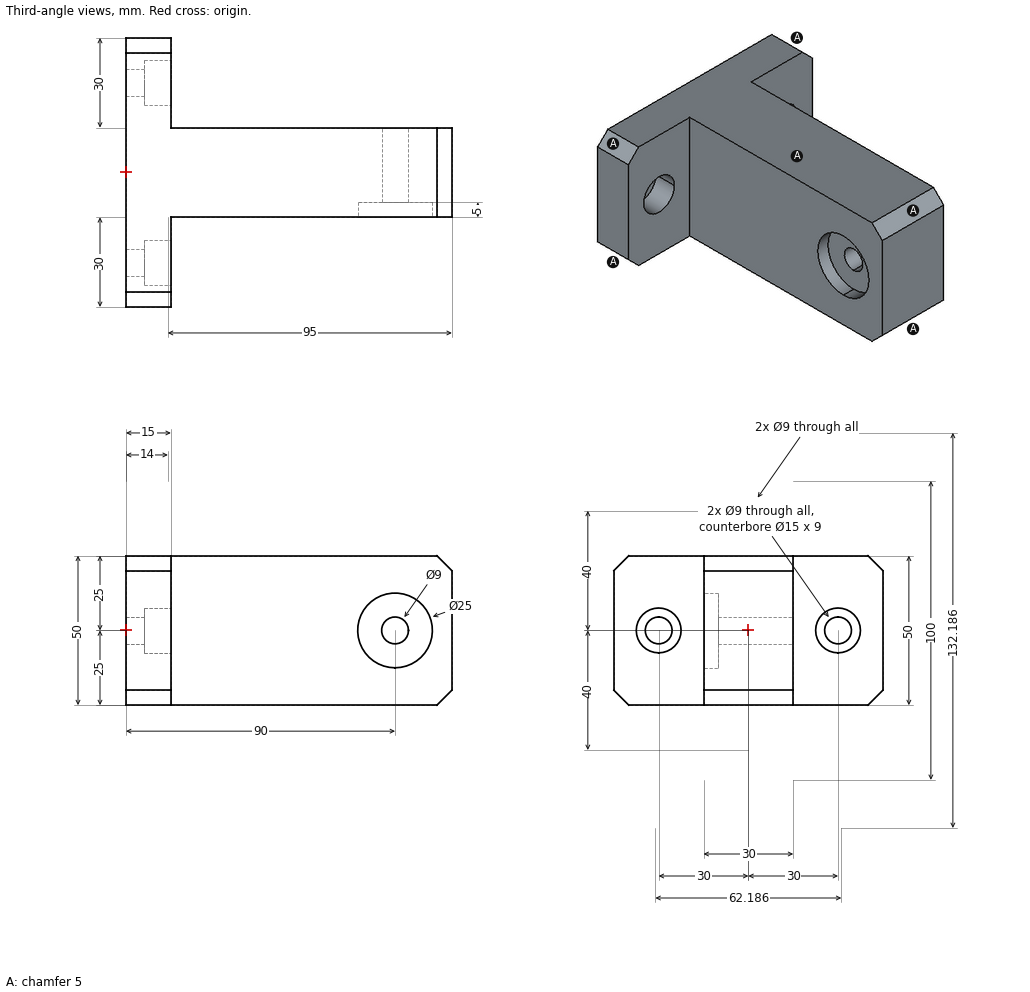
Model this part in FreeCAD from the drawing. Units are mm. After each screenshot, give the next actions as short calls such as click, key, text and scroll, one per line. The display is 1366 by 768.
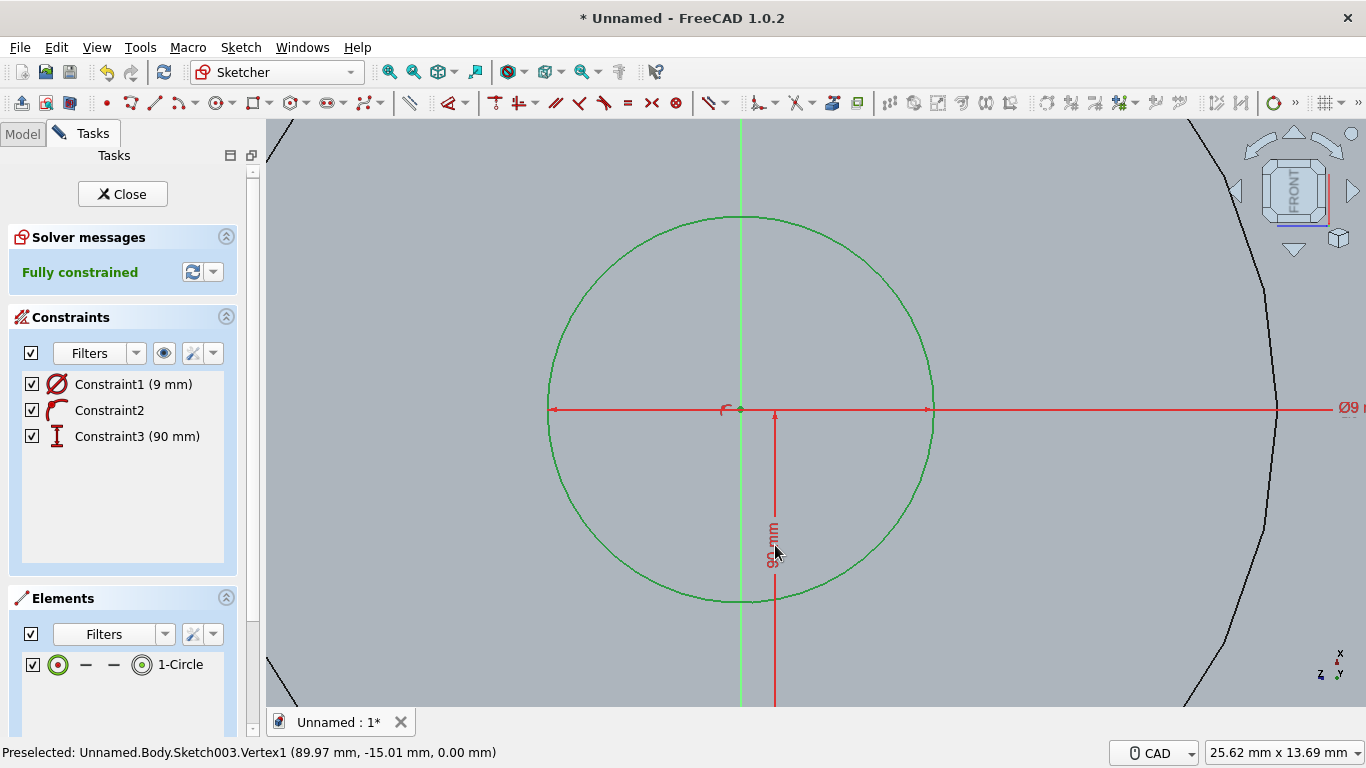
click(123, 194)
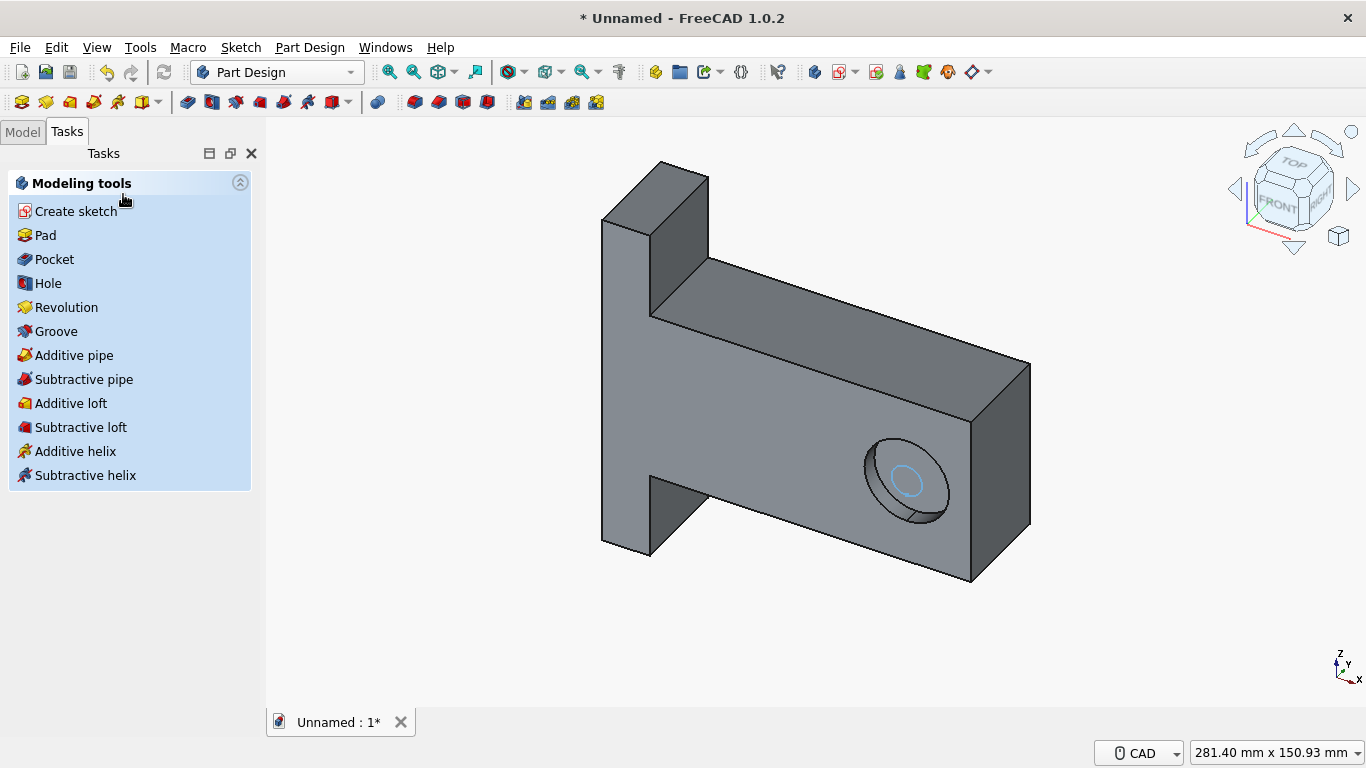
click(188, 102)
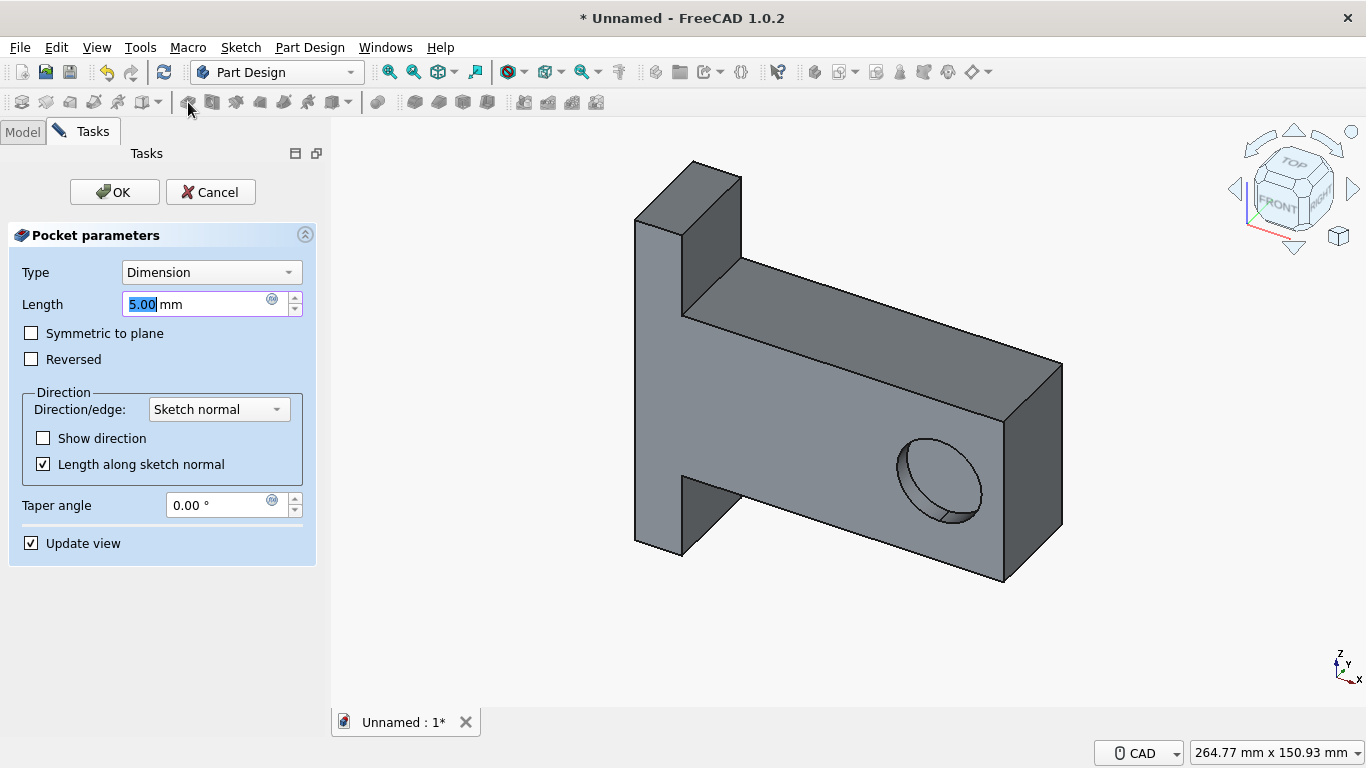
click(212, 272)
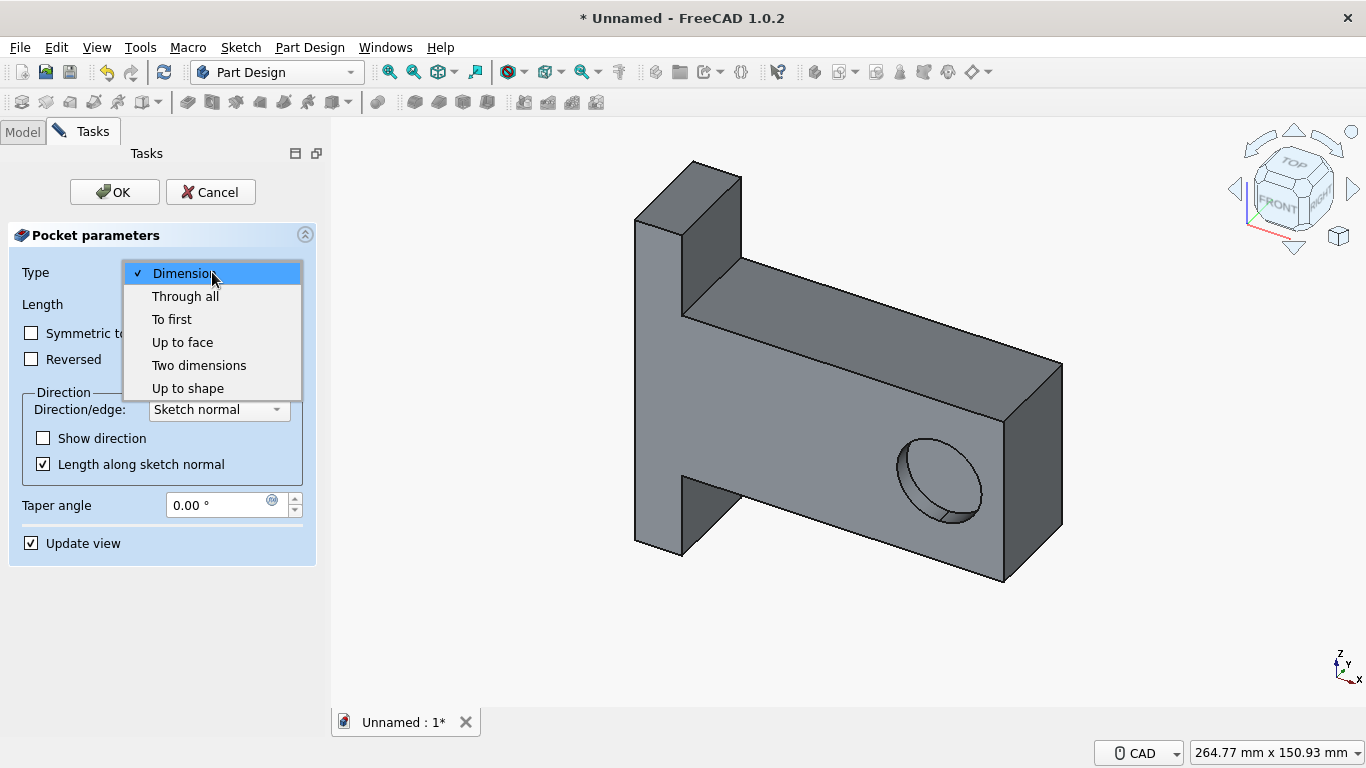
click(212, 296)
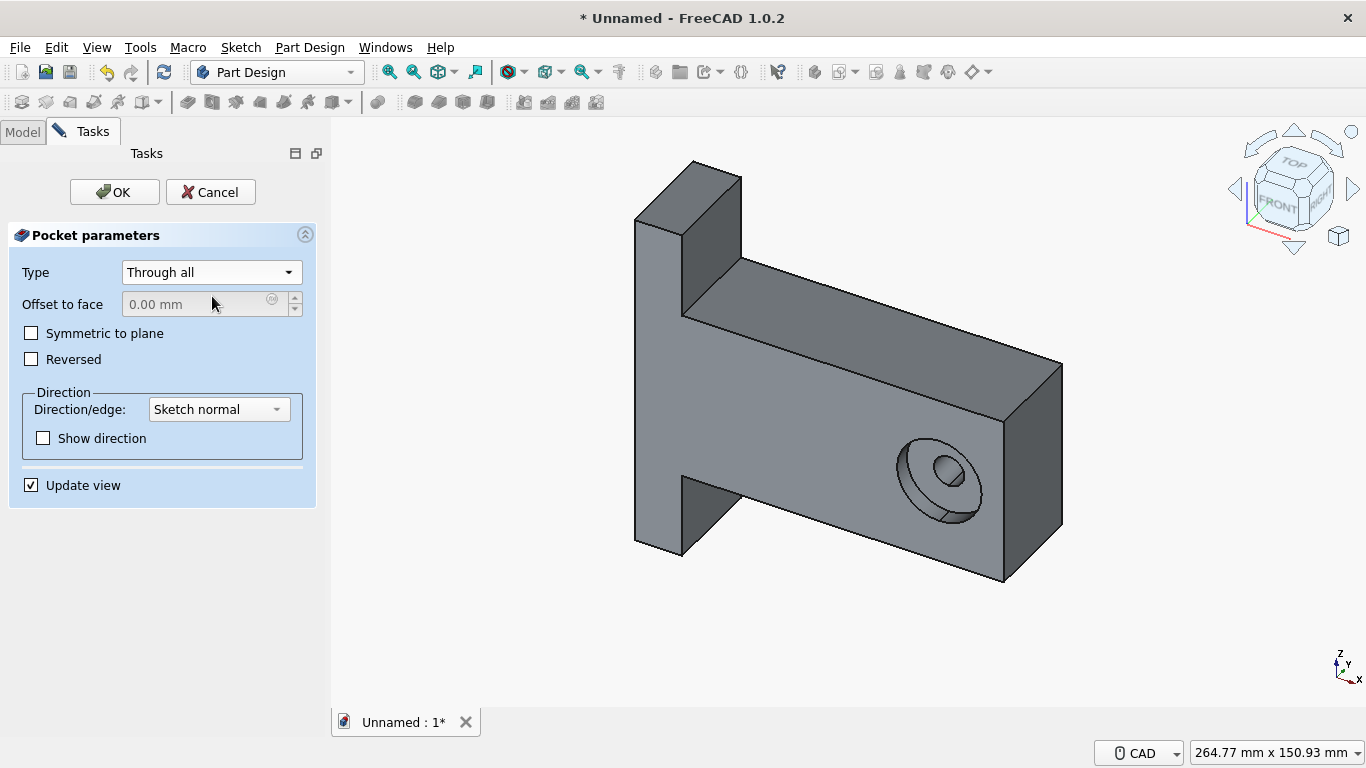
click(115, 192)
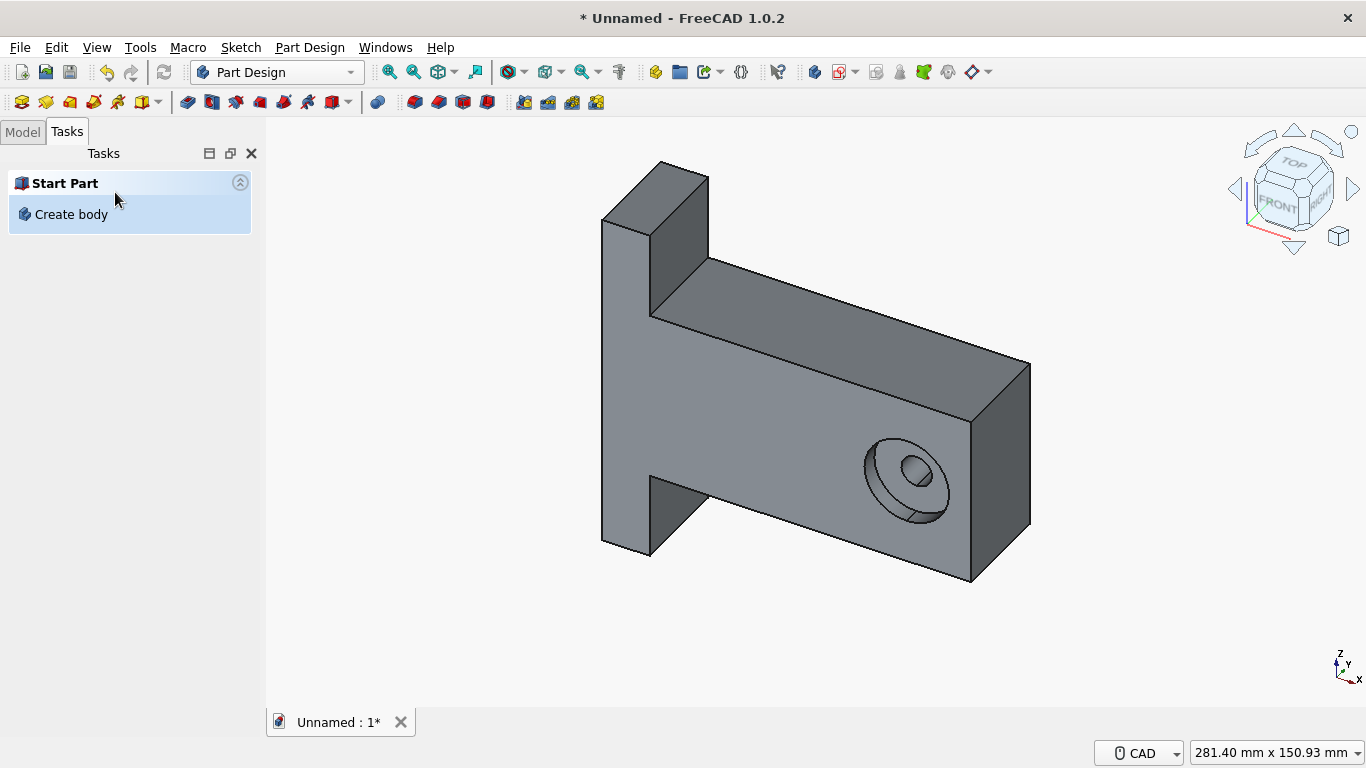
click(679, 246)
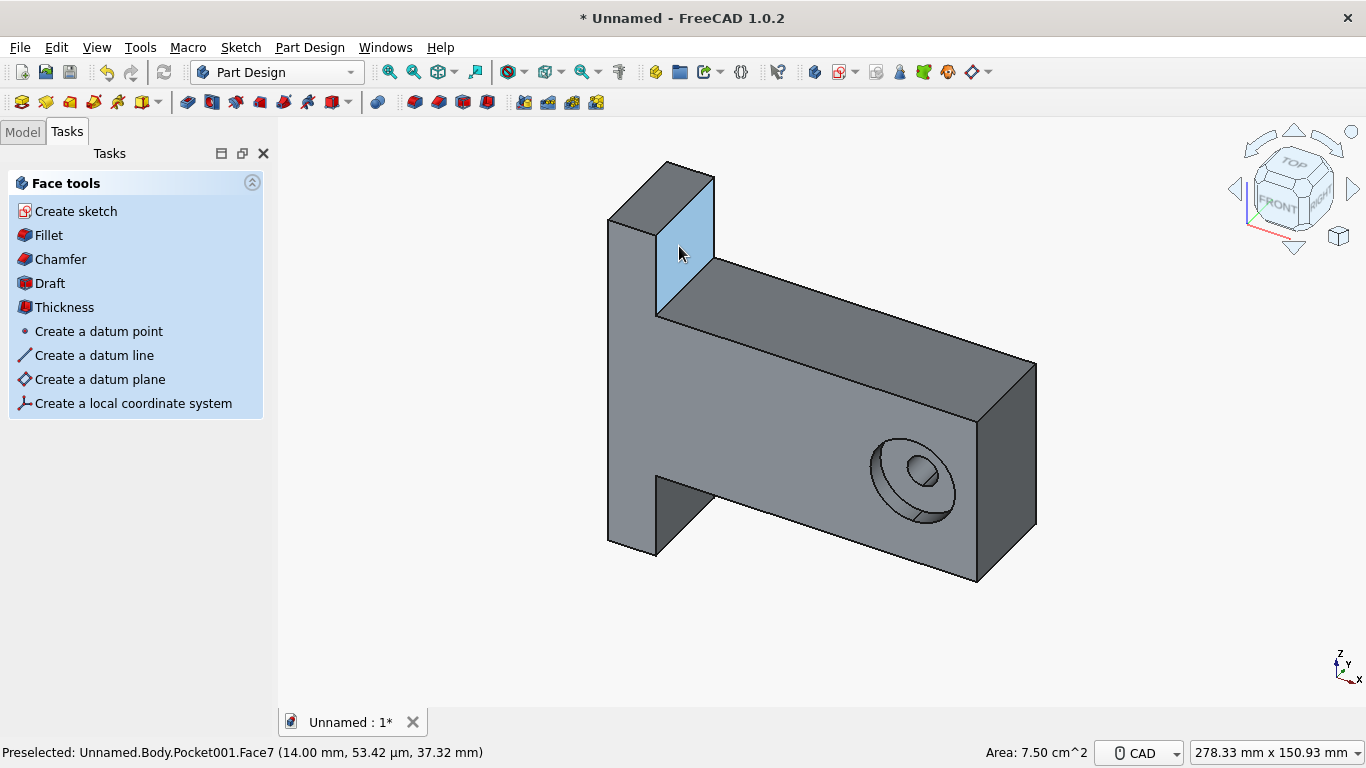
click(840, 72)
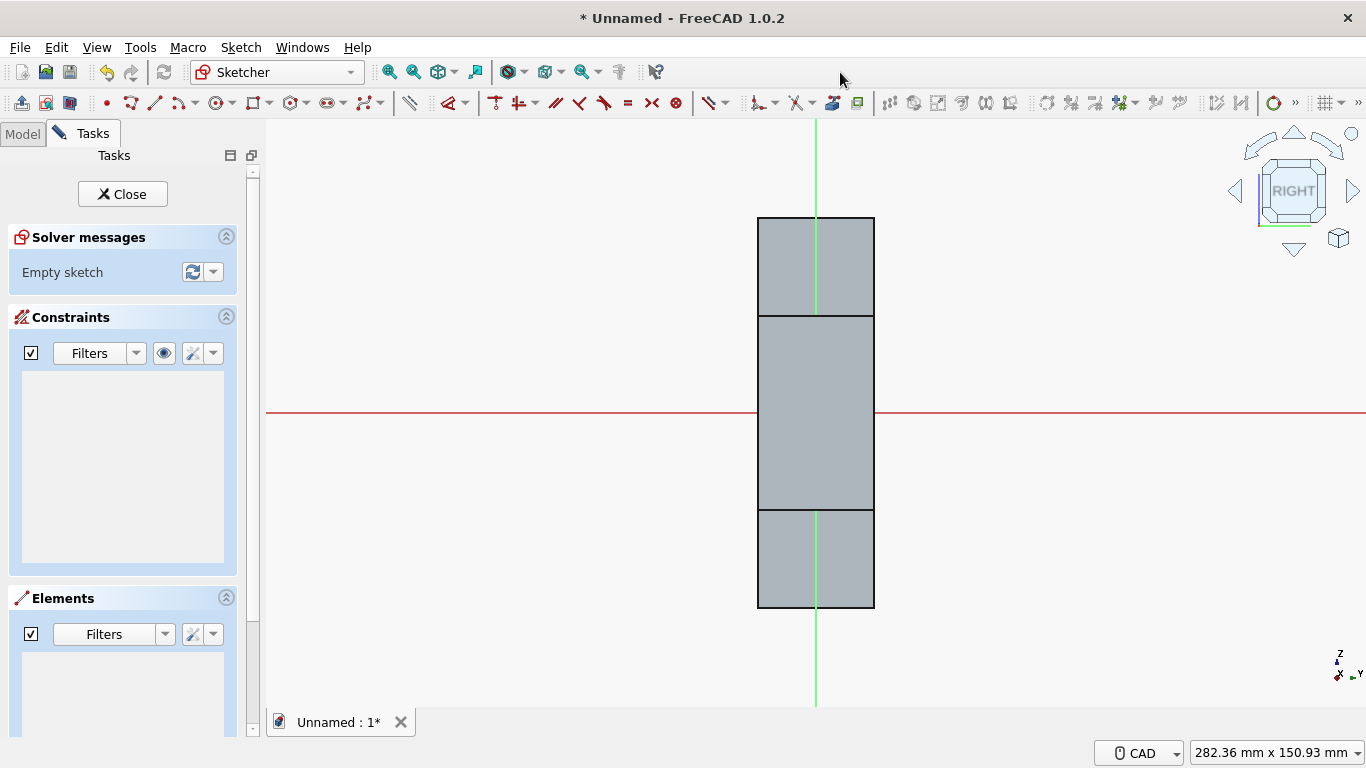
key(g)
key(c)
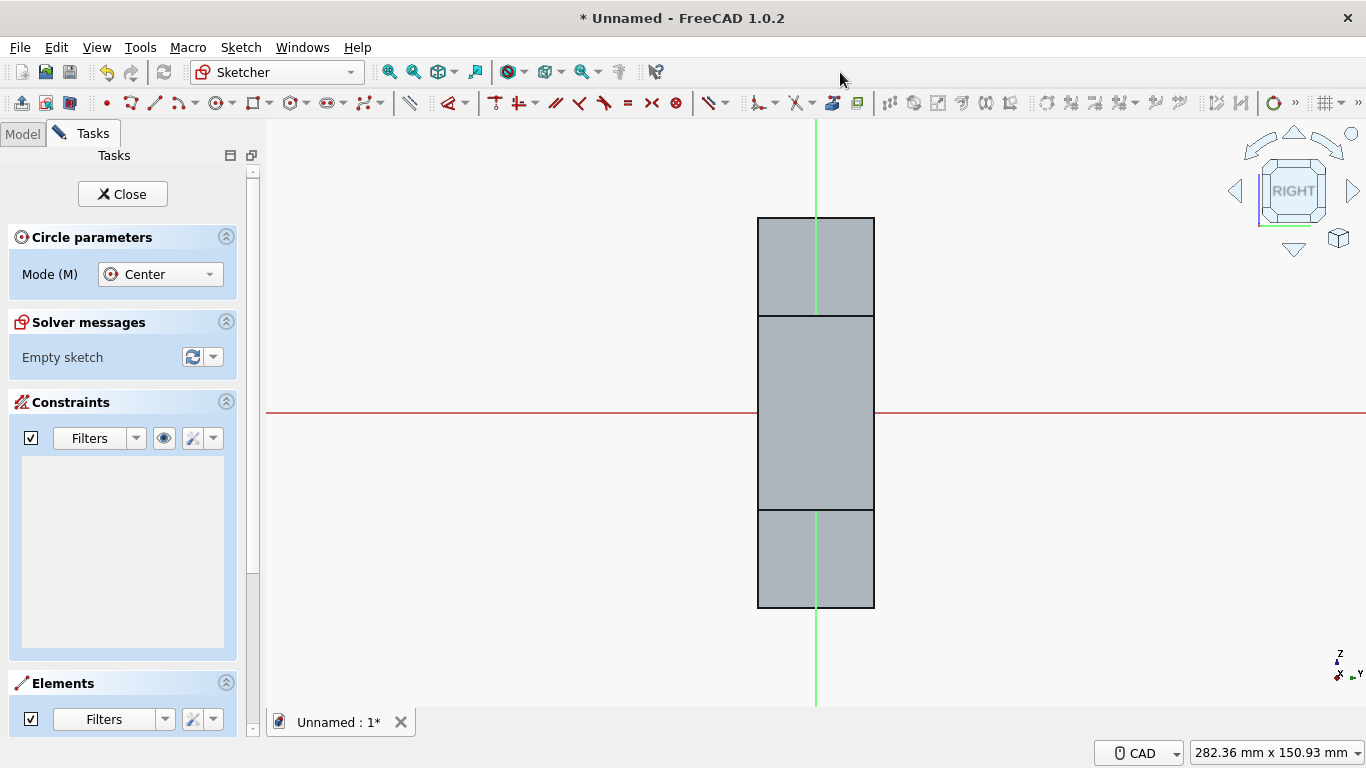
scroll(816, 257, up, 2)